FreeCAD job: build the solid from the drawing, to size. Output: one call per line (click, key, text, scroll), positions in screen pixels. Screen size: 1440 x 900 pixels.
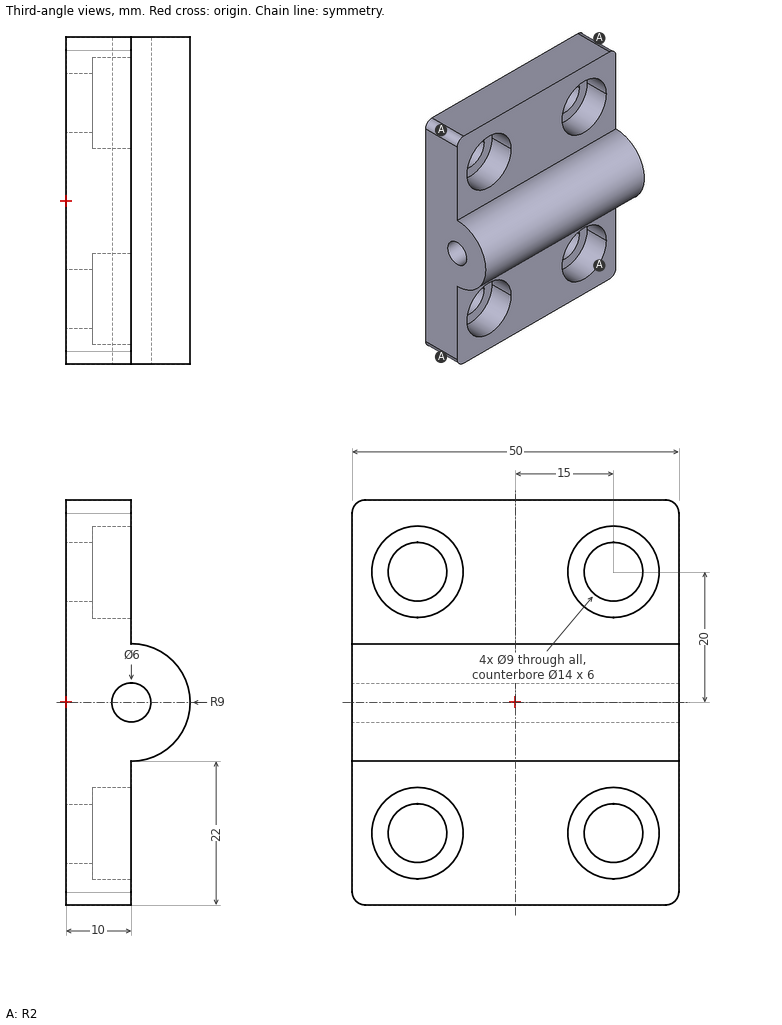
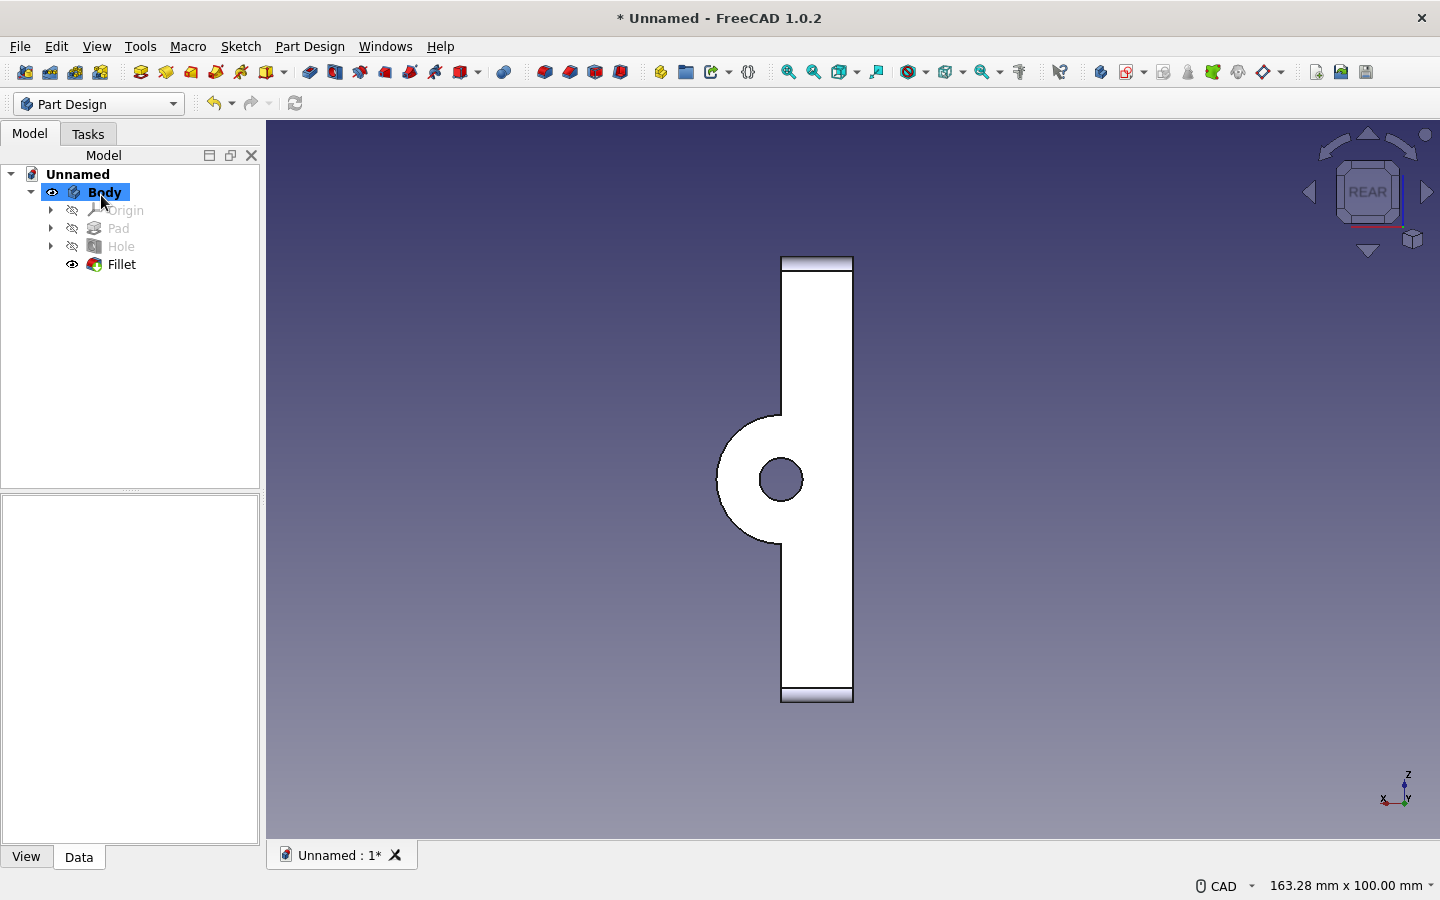
key(0)